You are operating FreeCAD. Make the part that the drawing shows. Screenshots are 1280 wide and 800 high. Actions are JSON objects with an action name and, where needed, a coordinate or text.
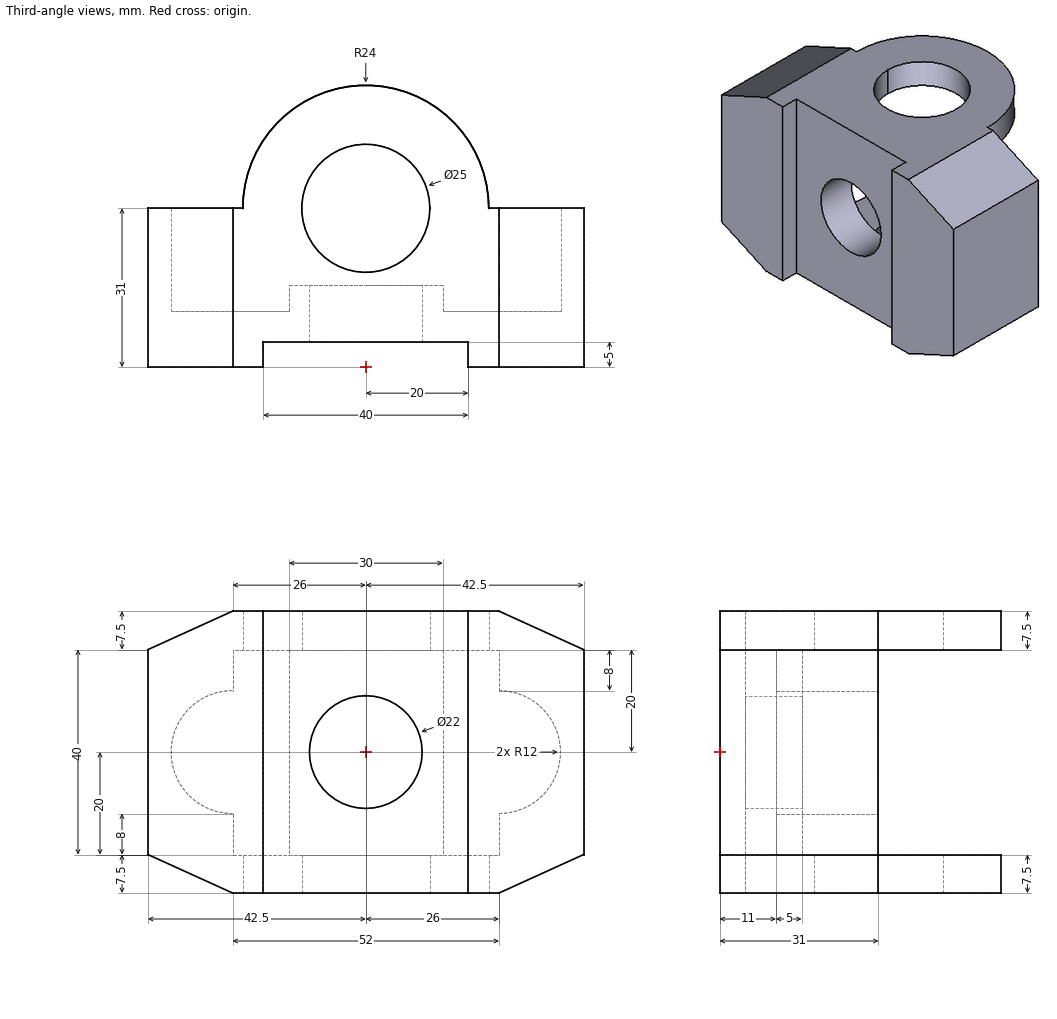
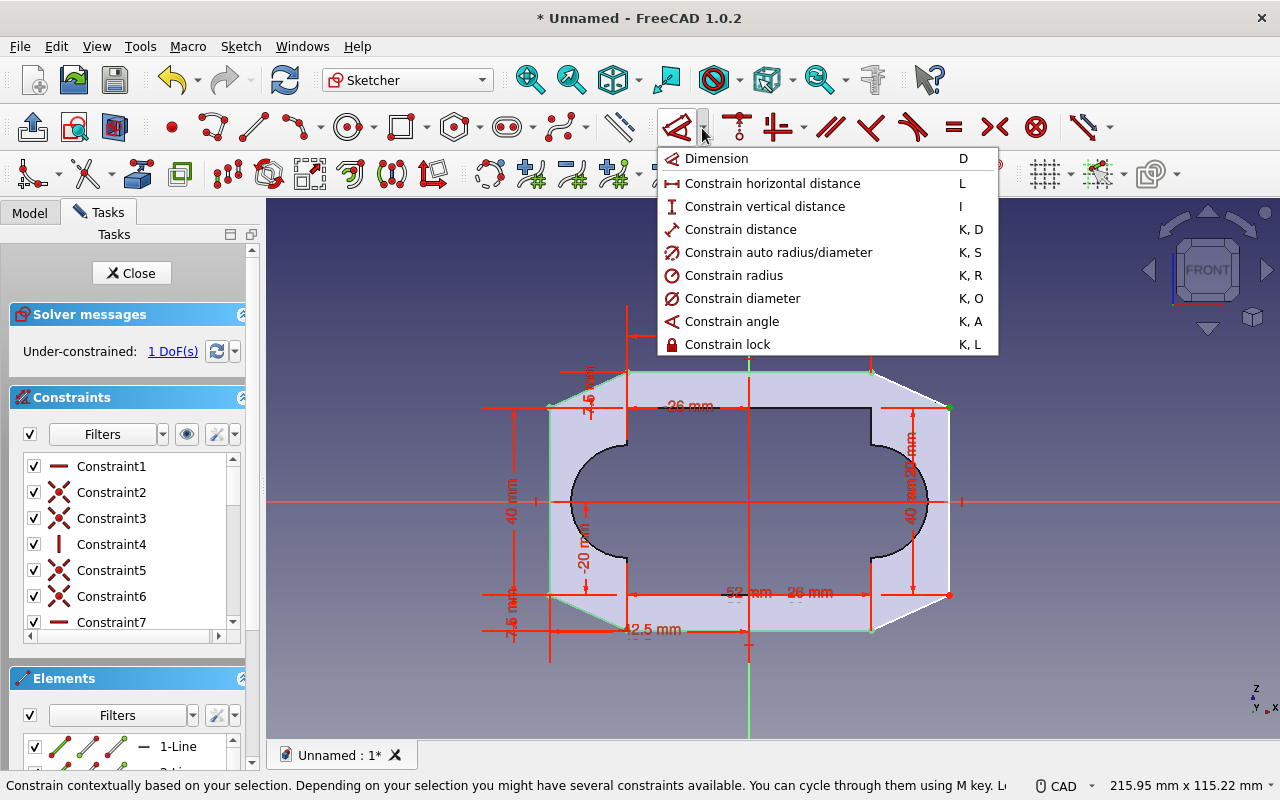
{"action": "left_click", "coordinate": [828, 184]}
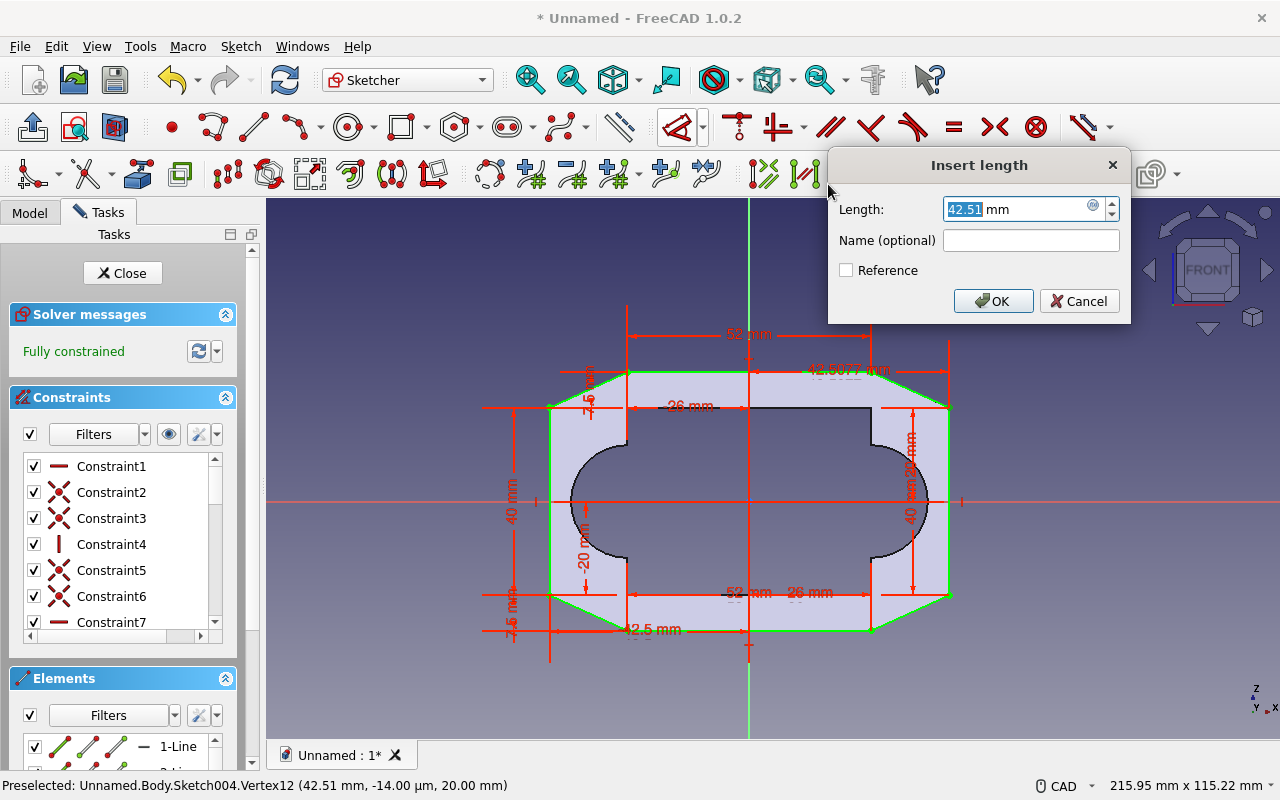
{"action": "type", "text": "42.5"}
{"action": "key", "text": "Return"}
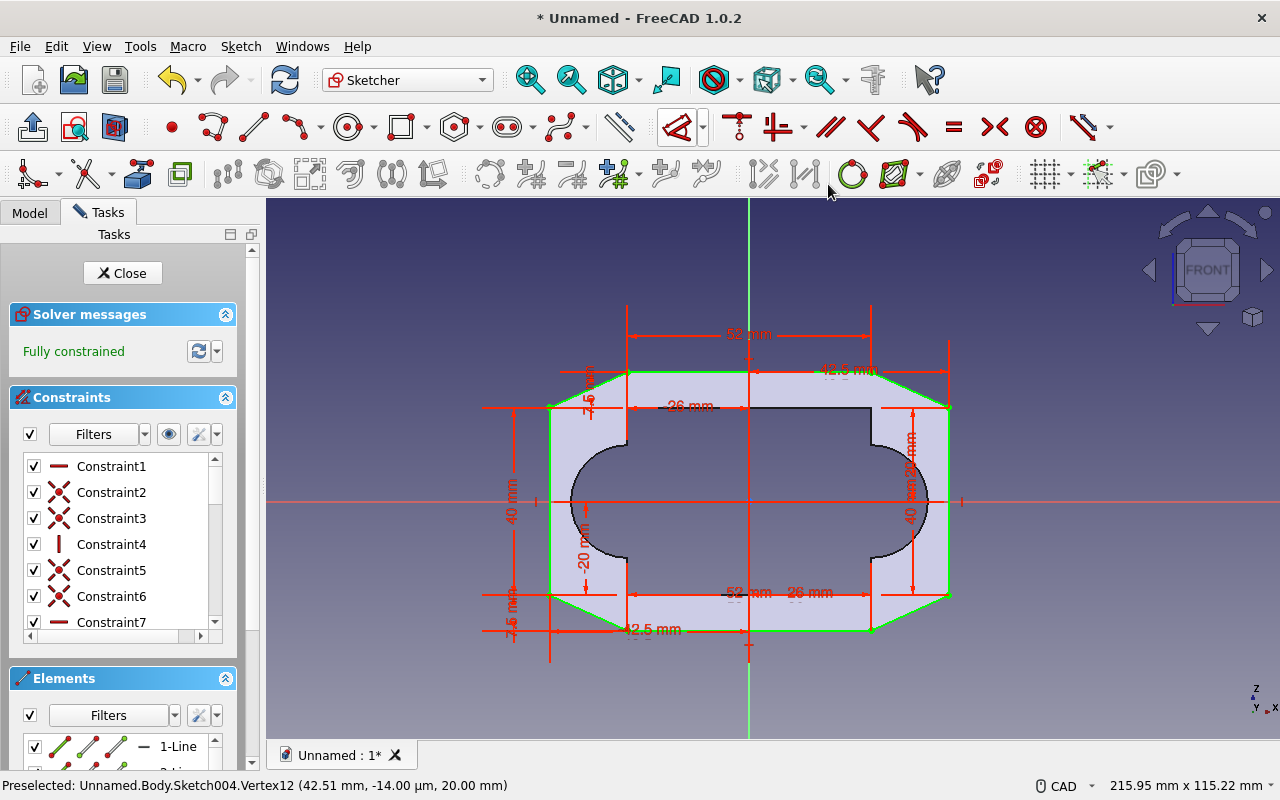
{"action": "left_click", "coordinate": [123, 273]}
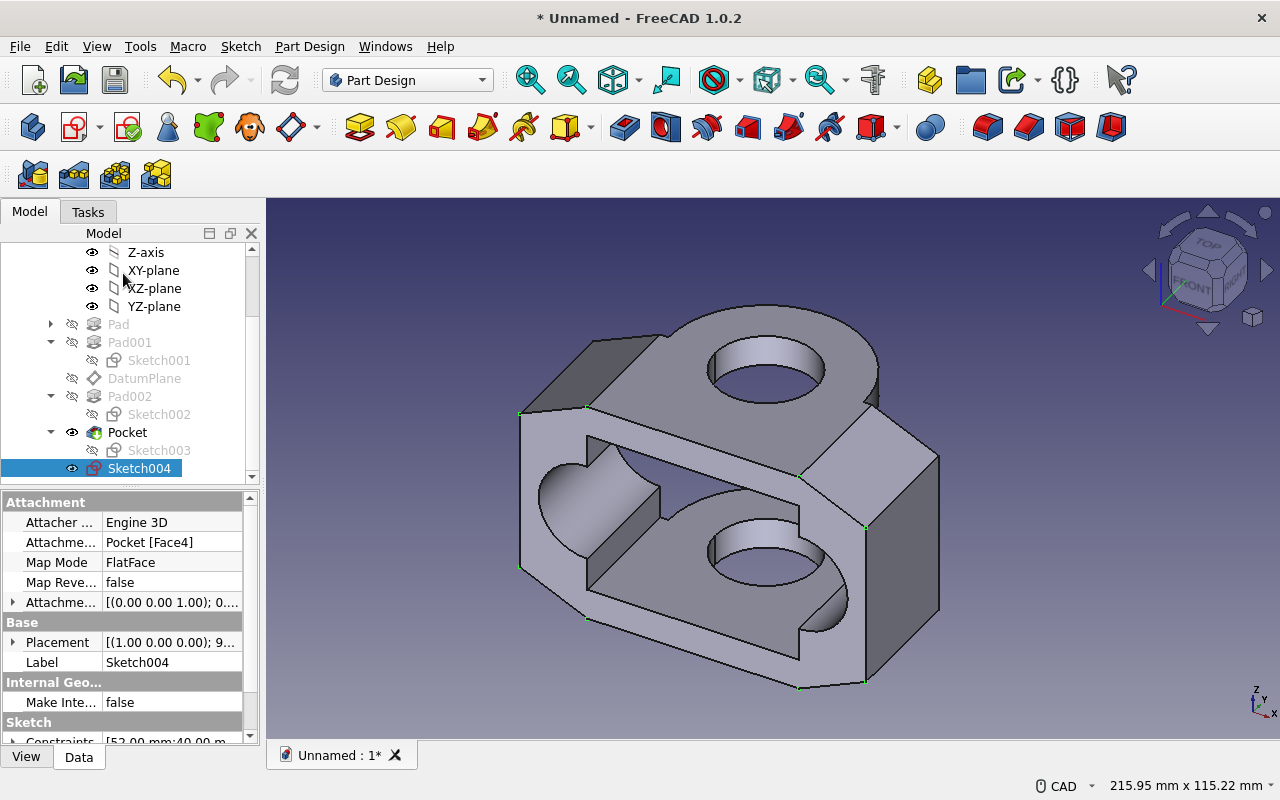
{"action": "left_click", "coordinate": [360, 128]}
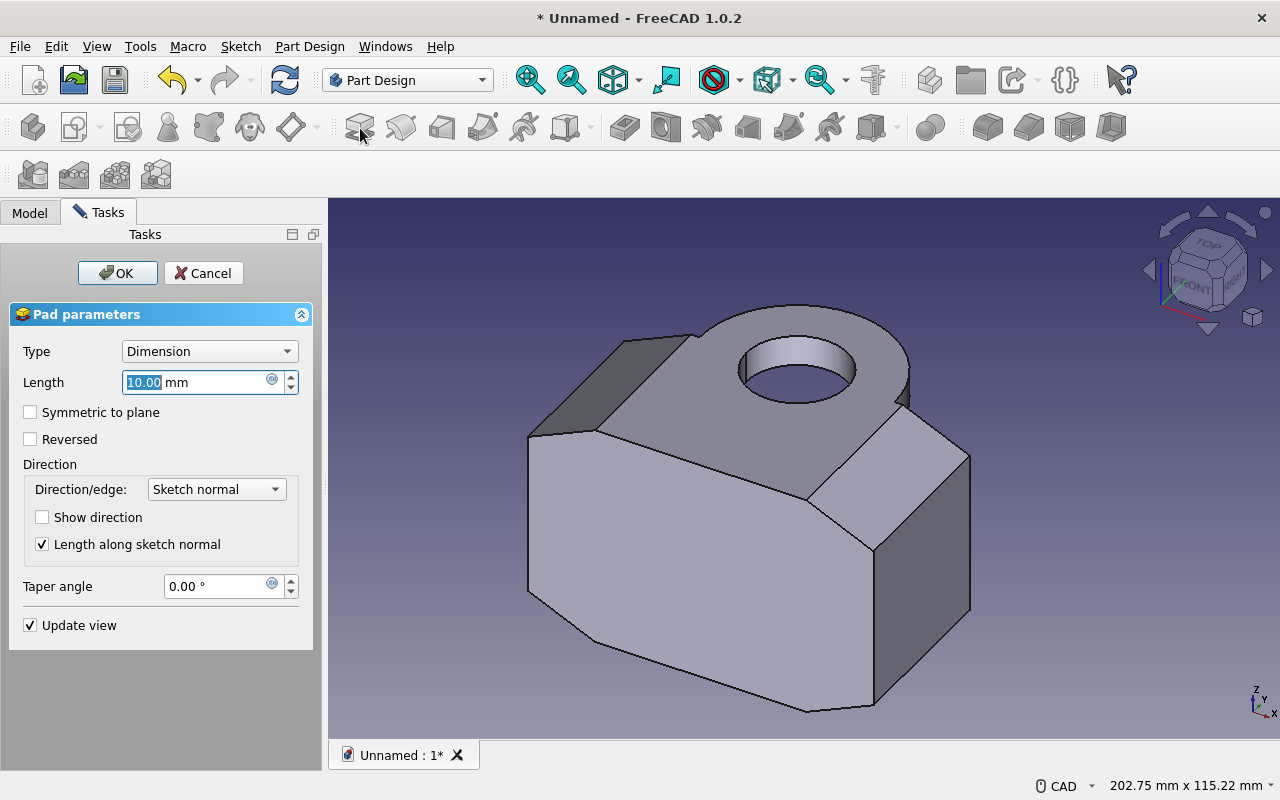
{"action": "type", "text": "11"}
{"action": "key", "text": "Tab"}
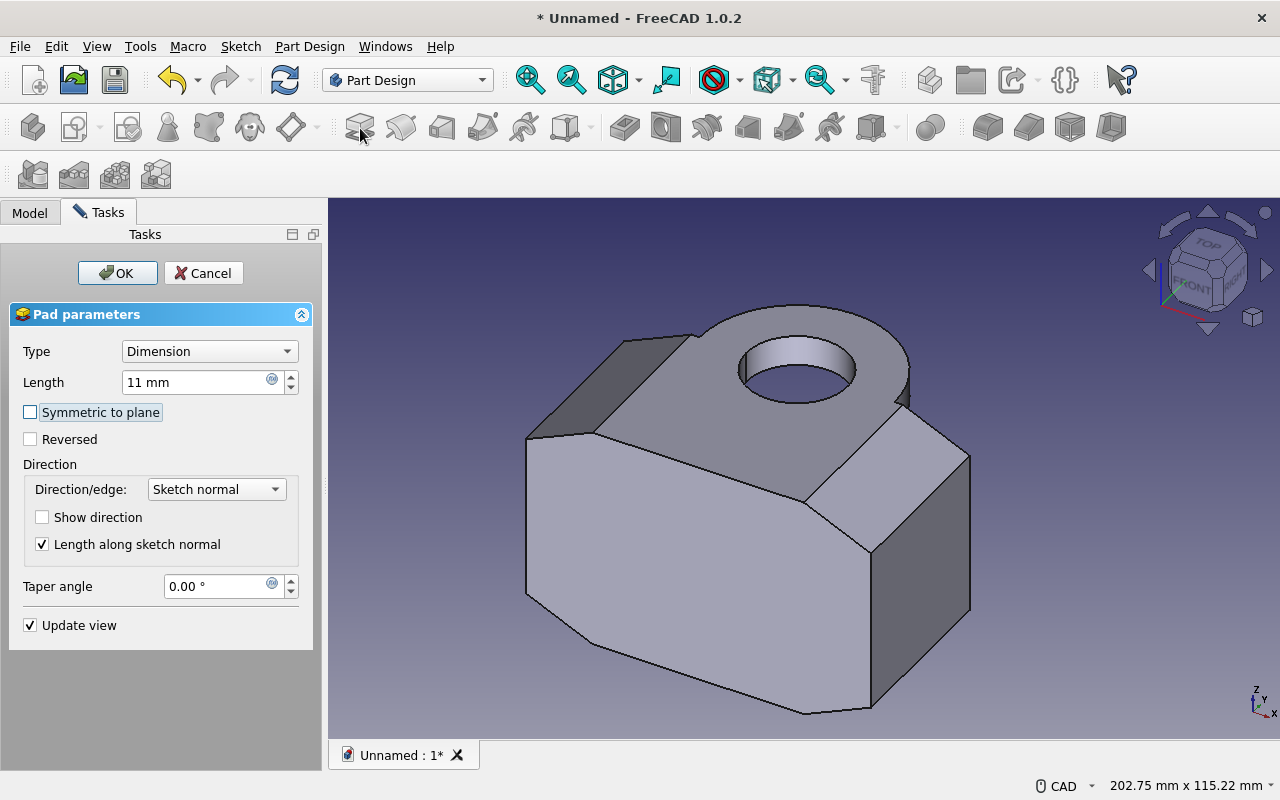
{"action": "left_click", "coordinate": [31, 439]}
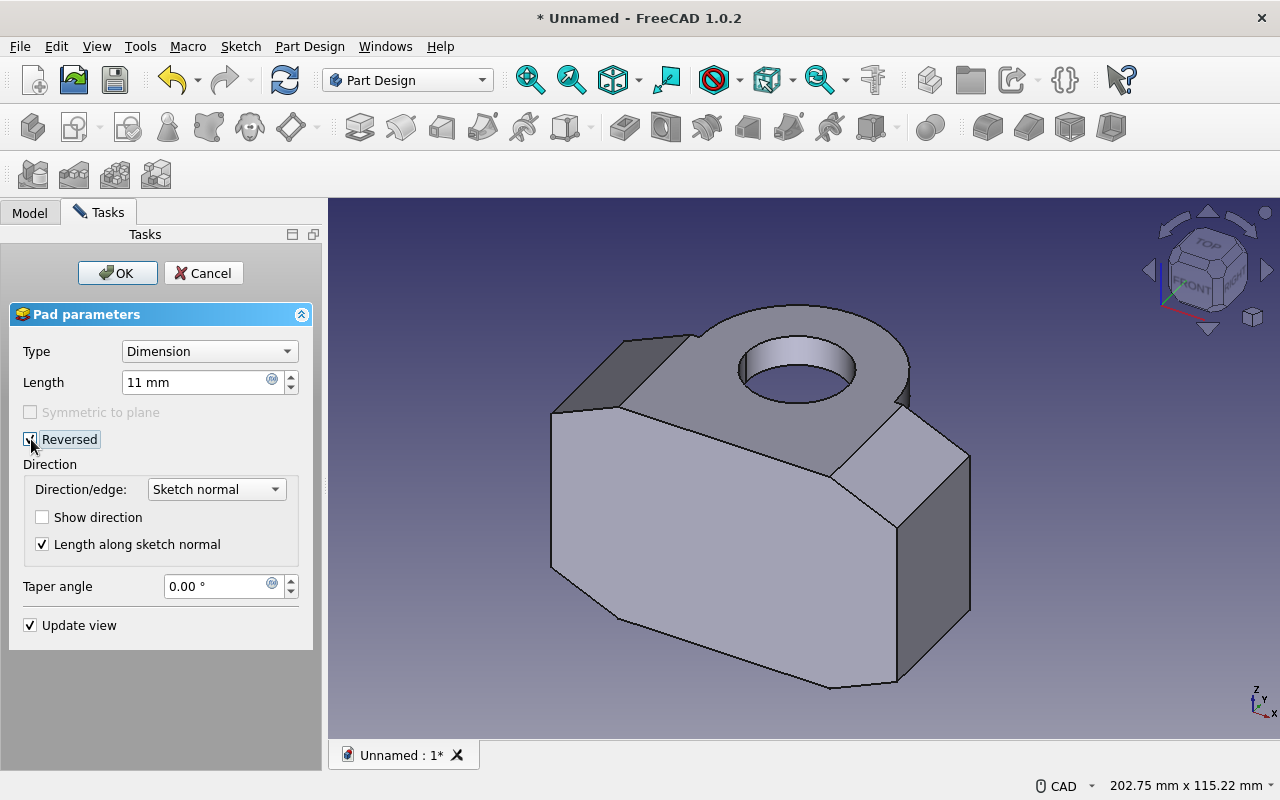
{"action": "left_click", "coordinate": [118, 273]}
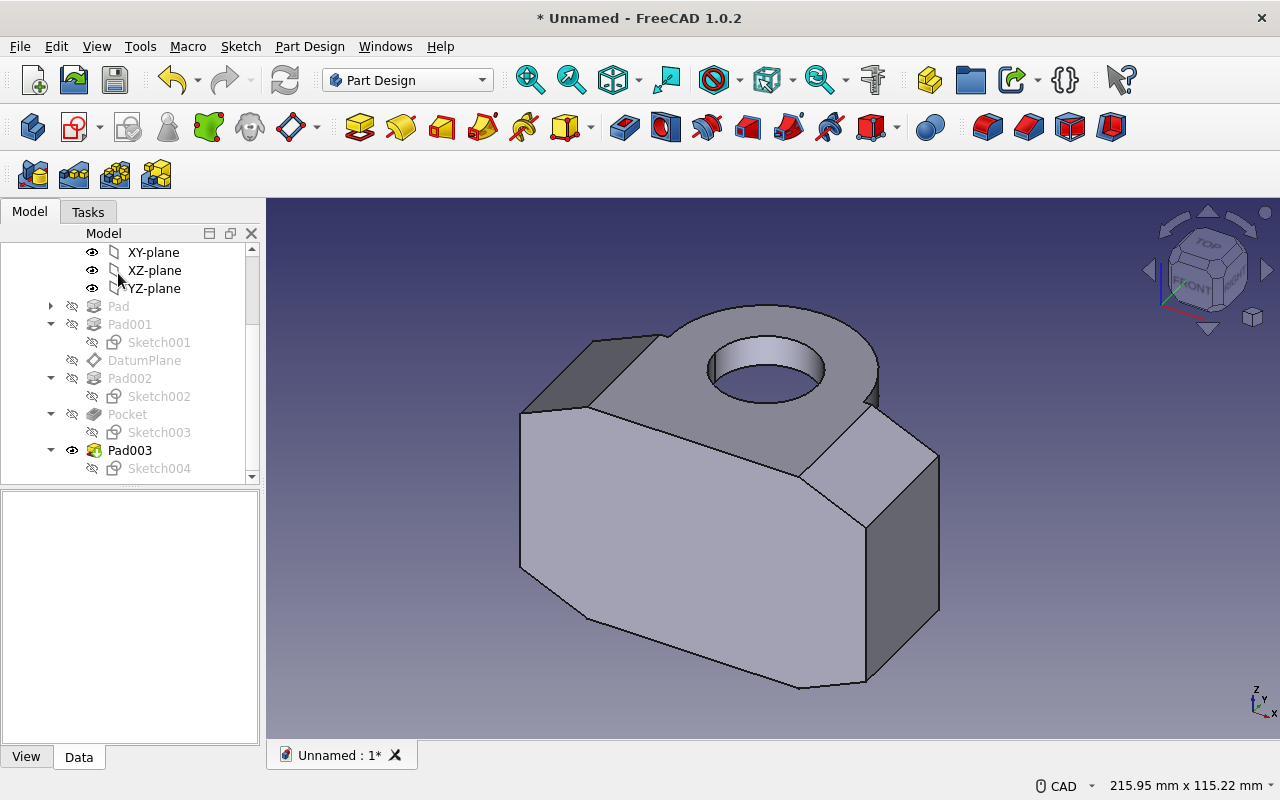
{"action": "key", "text": "4"}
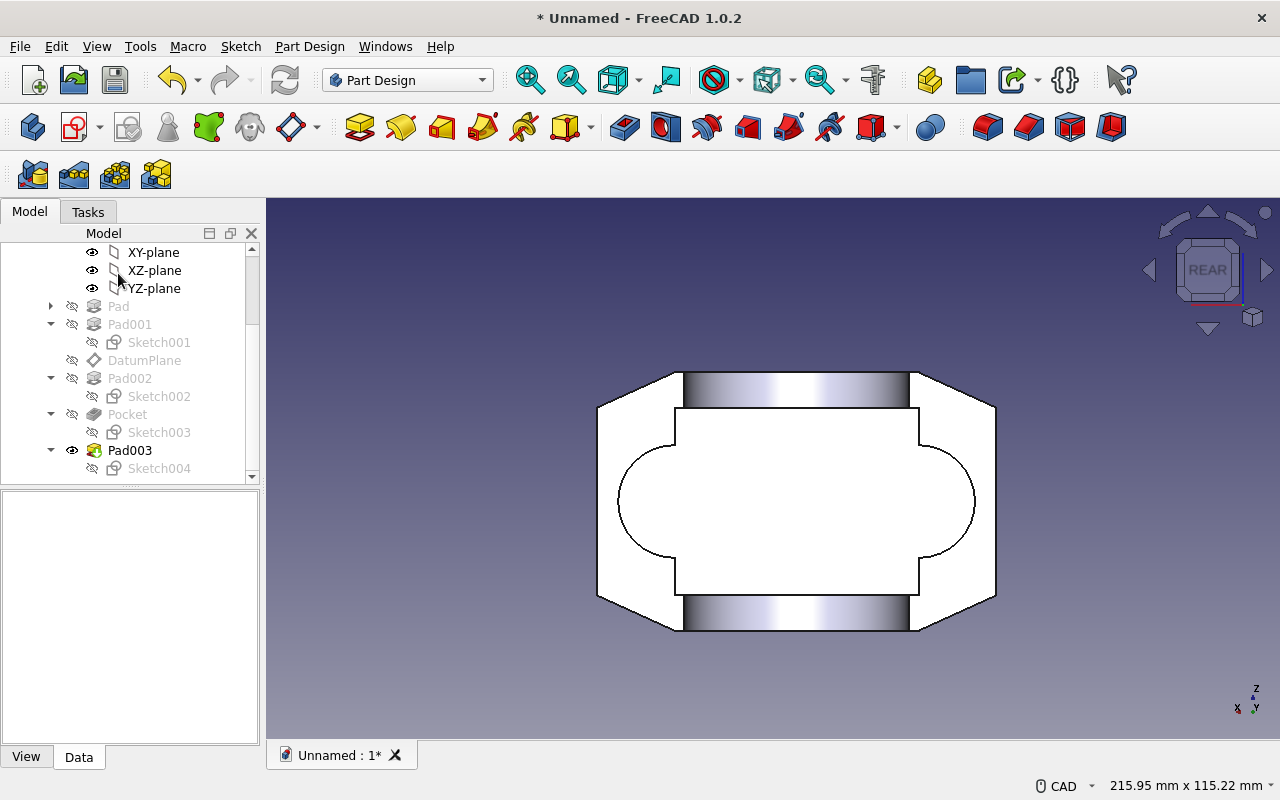
{"action": "left_click", "coordinate": [797, 501]}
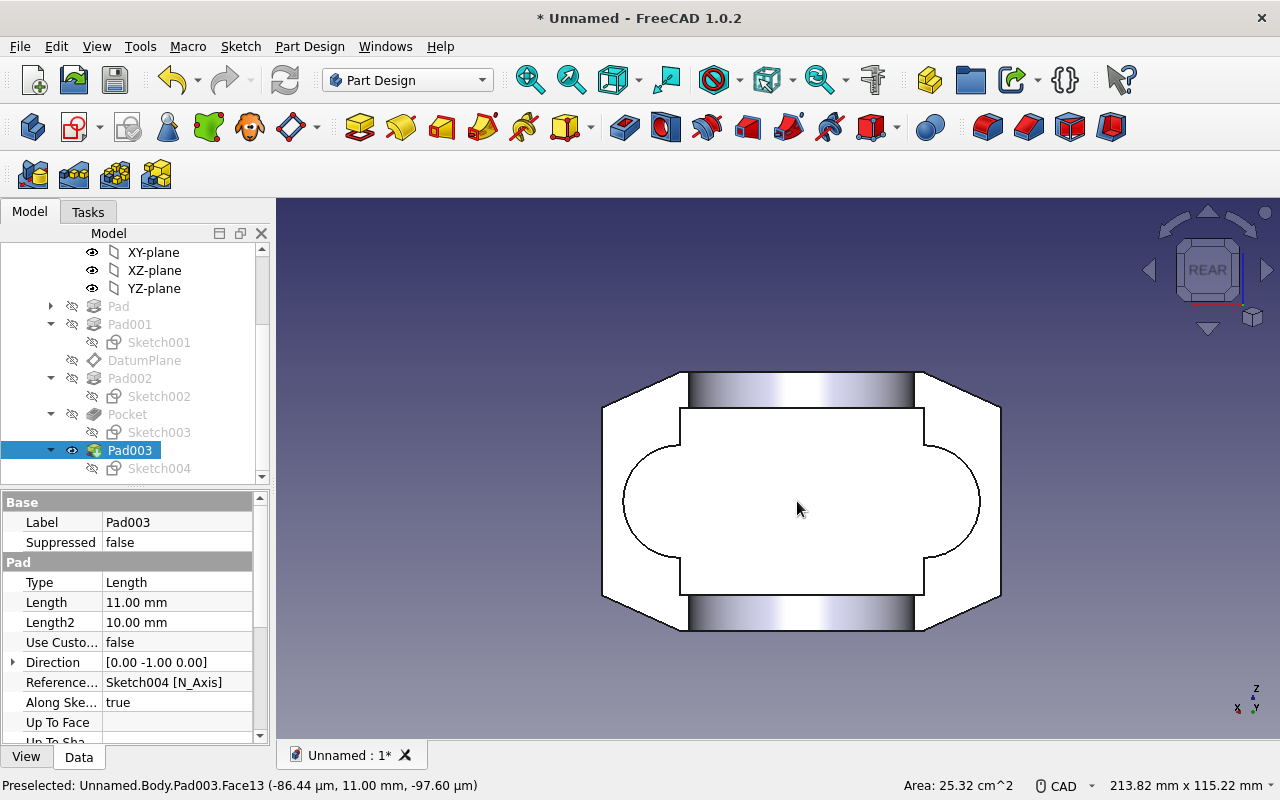
{"action": "left_click", "coordinate": [74, 128]}